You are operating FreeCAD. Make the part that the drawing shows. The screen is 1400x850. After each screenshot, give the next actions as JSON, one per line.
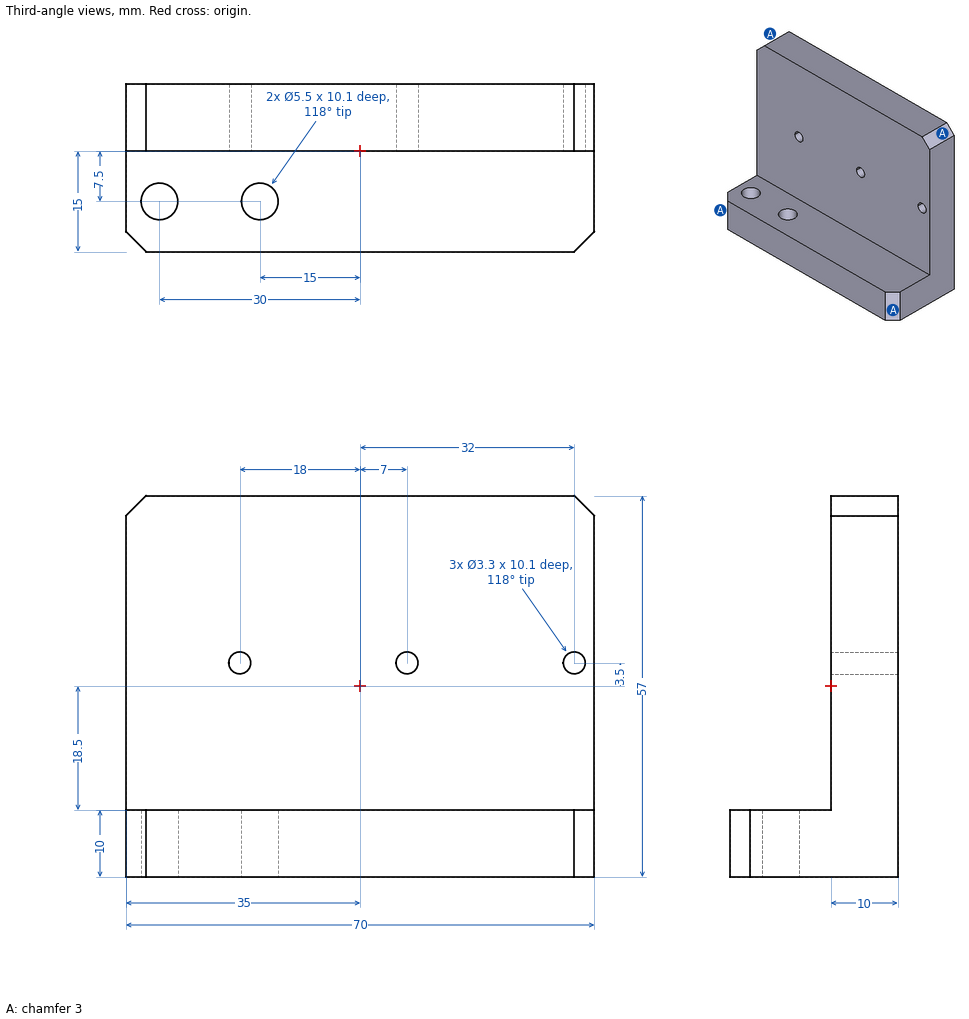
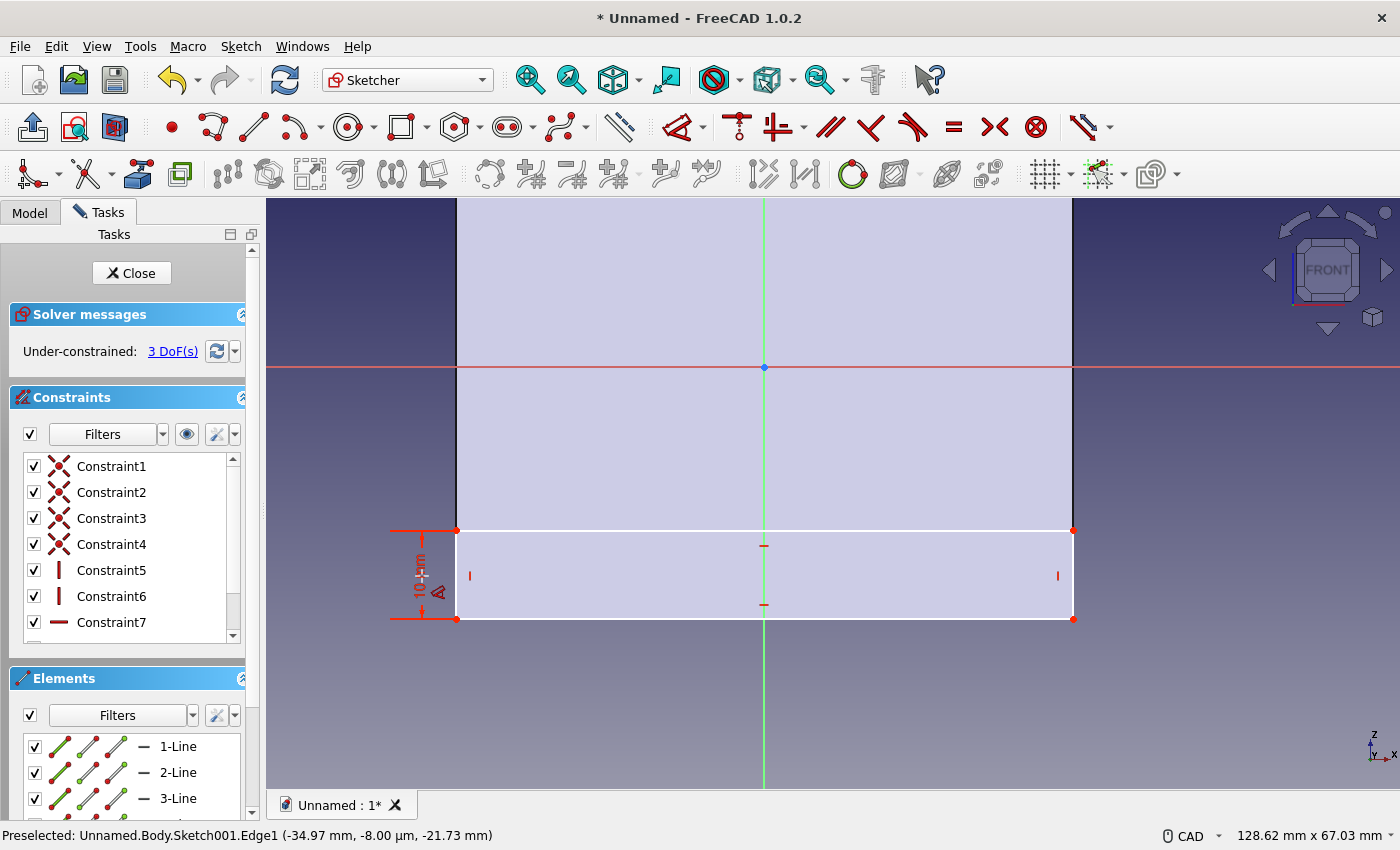
{"action": "left_click", "coordinate": [641, 619]}
{"action": "left_click", "coordinate": [623, 653]}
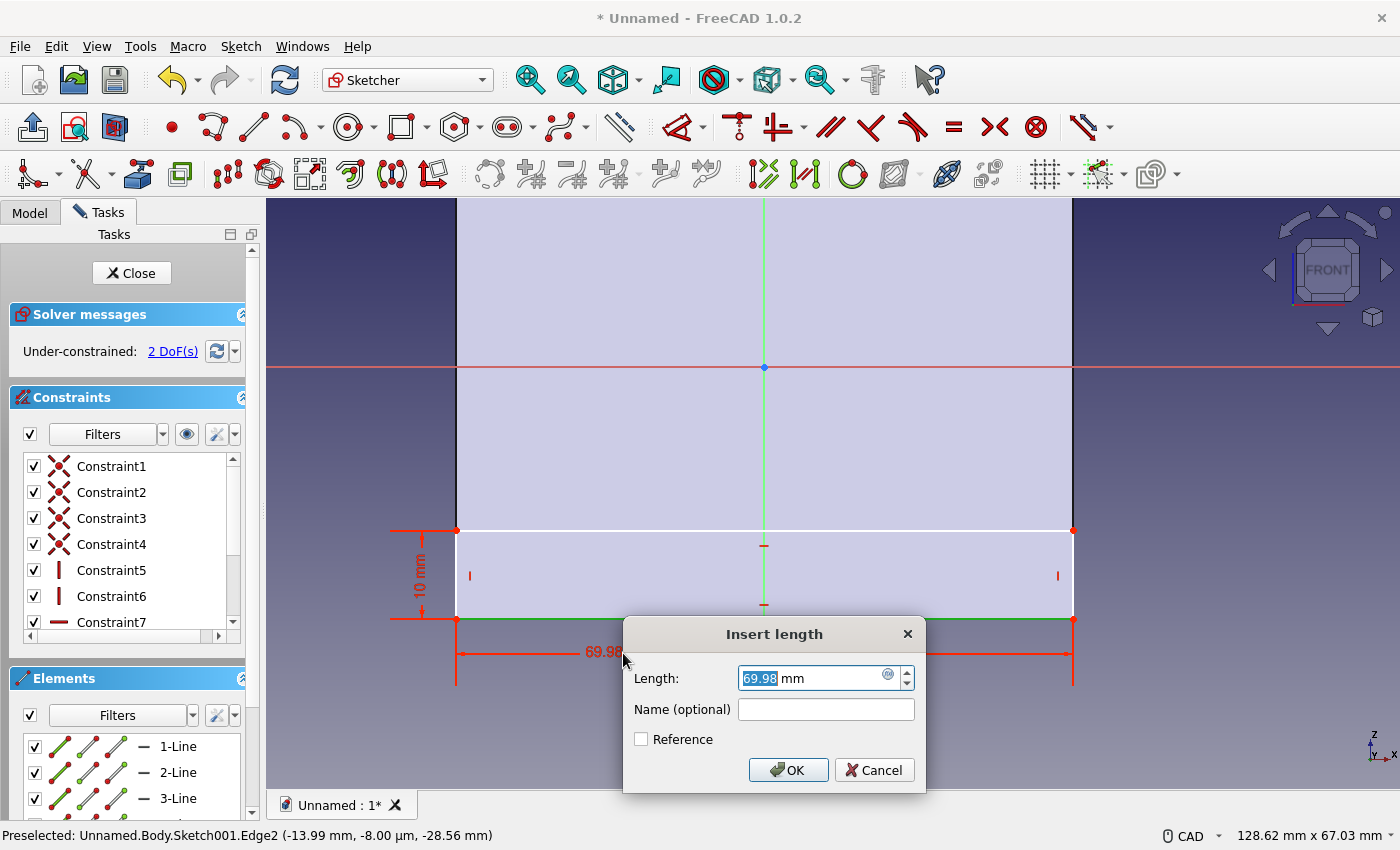
{"action": "type", "text": "70"}
{"action": "key", "text": "Return"}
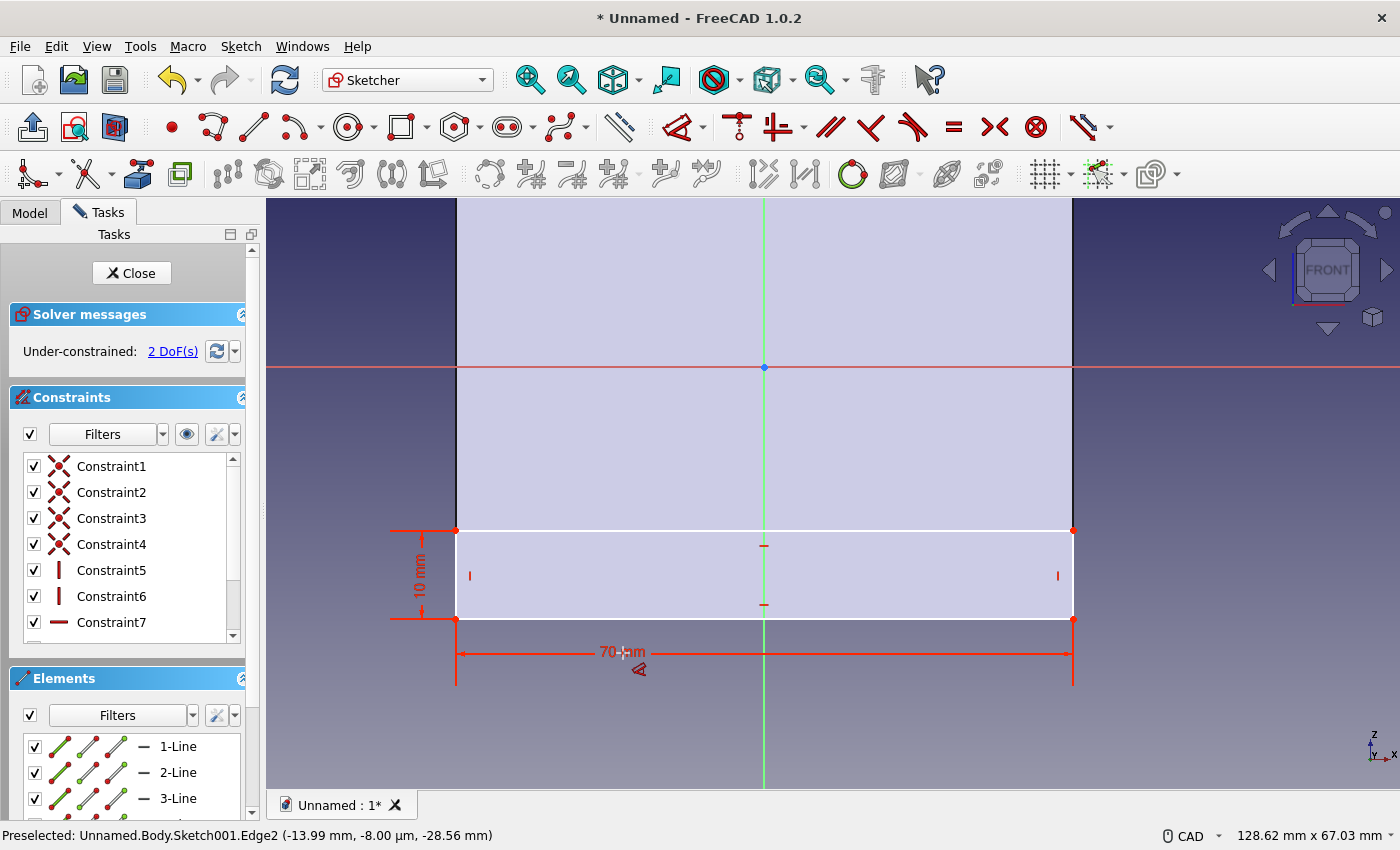
{"action": "left_click", "coordinate": [456, 531]}
{"action": "left_click", "coordinate": [610, 333]}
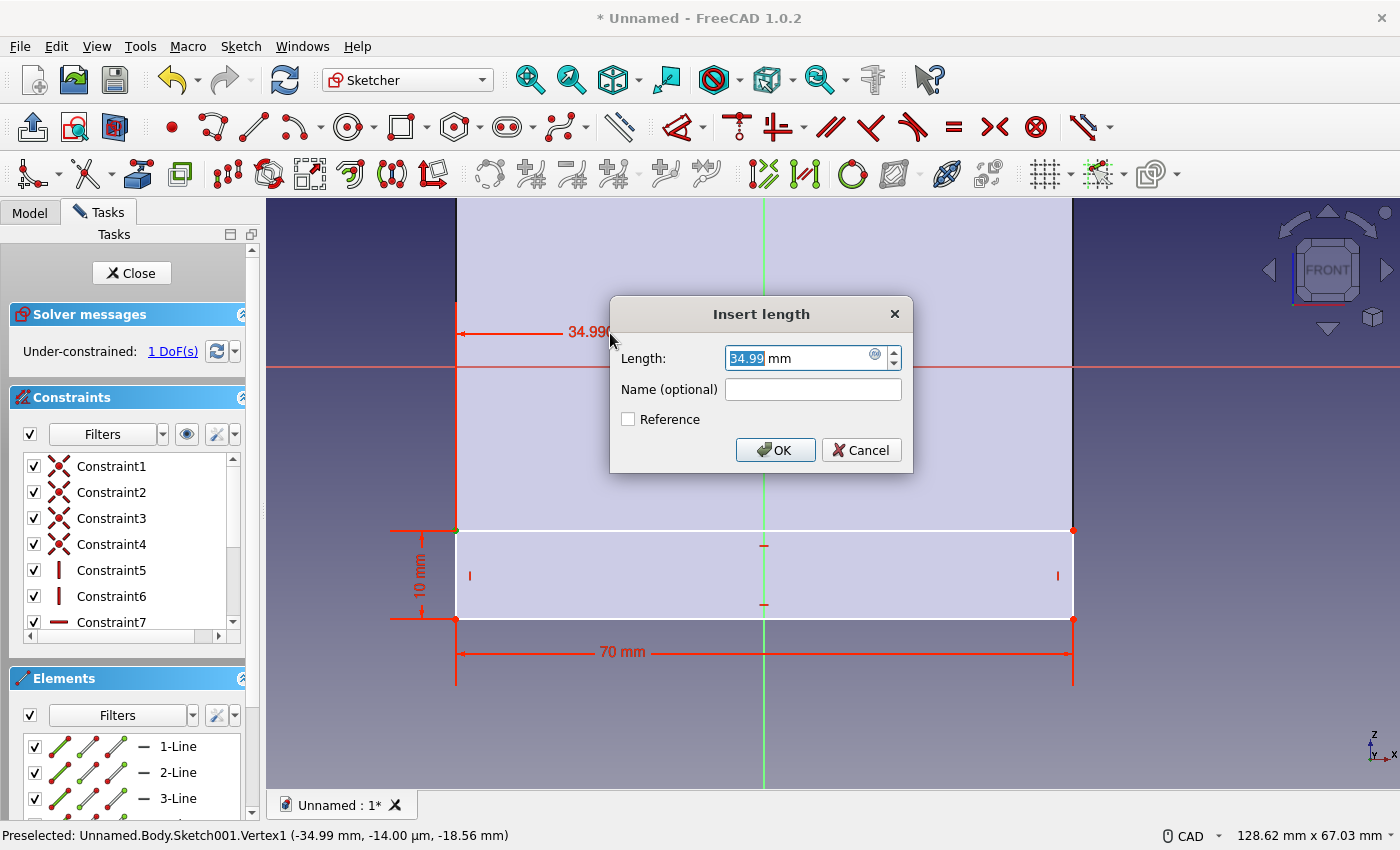
{"action": "type", "text": "35"}
{"action": "key", "text": "Return"}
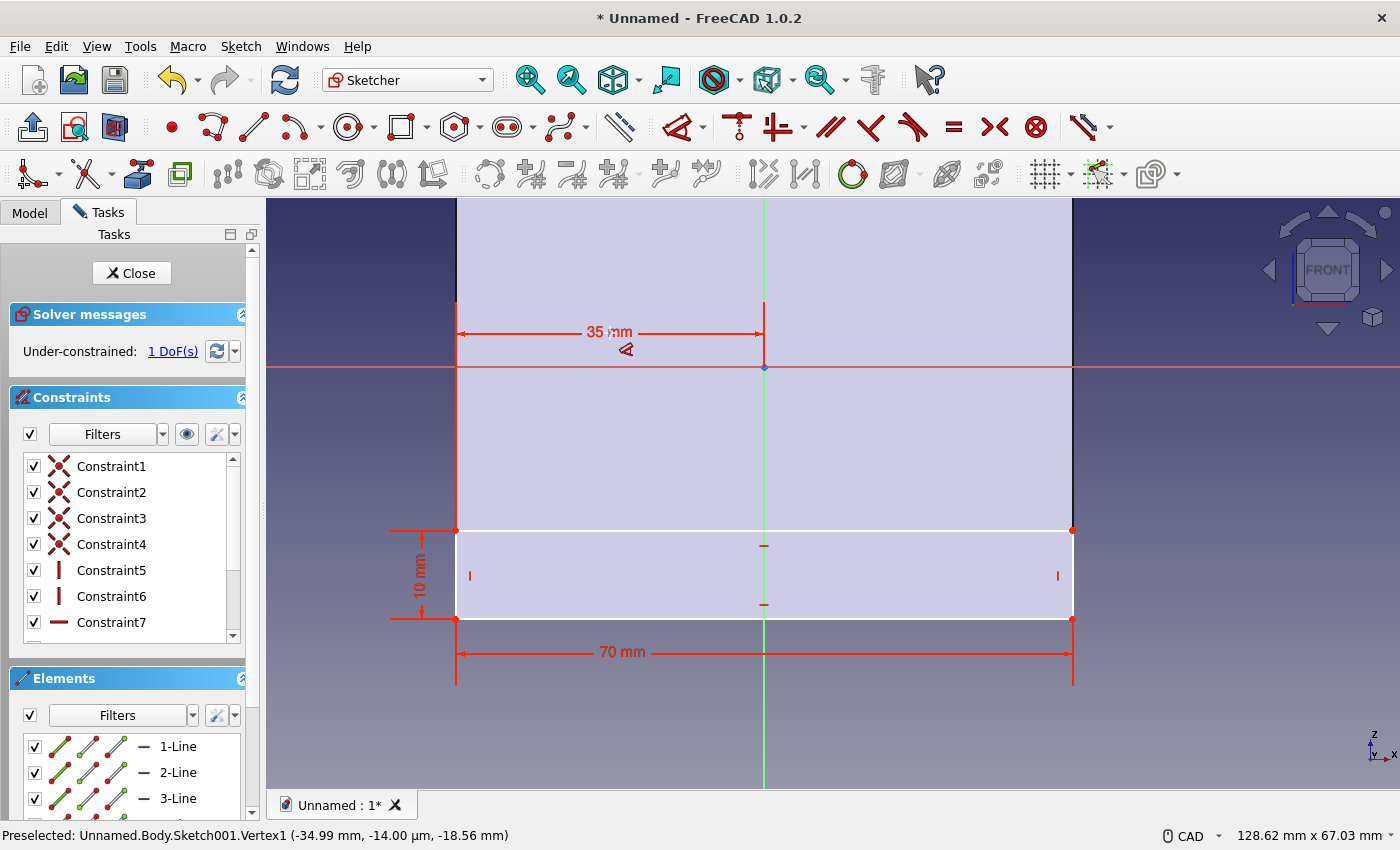
{"action": "left_click", "coordinate": [456, 531]}
{"action": "left_click", "coordinate": [422, 449]}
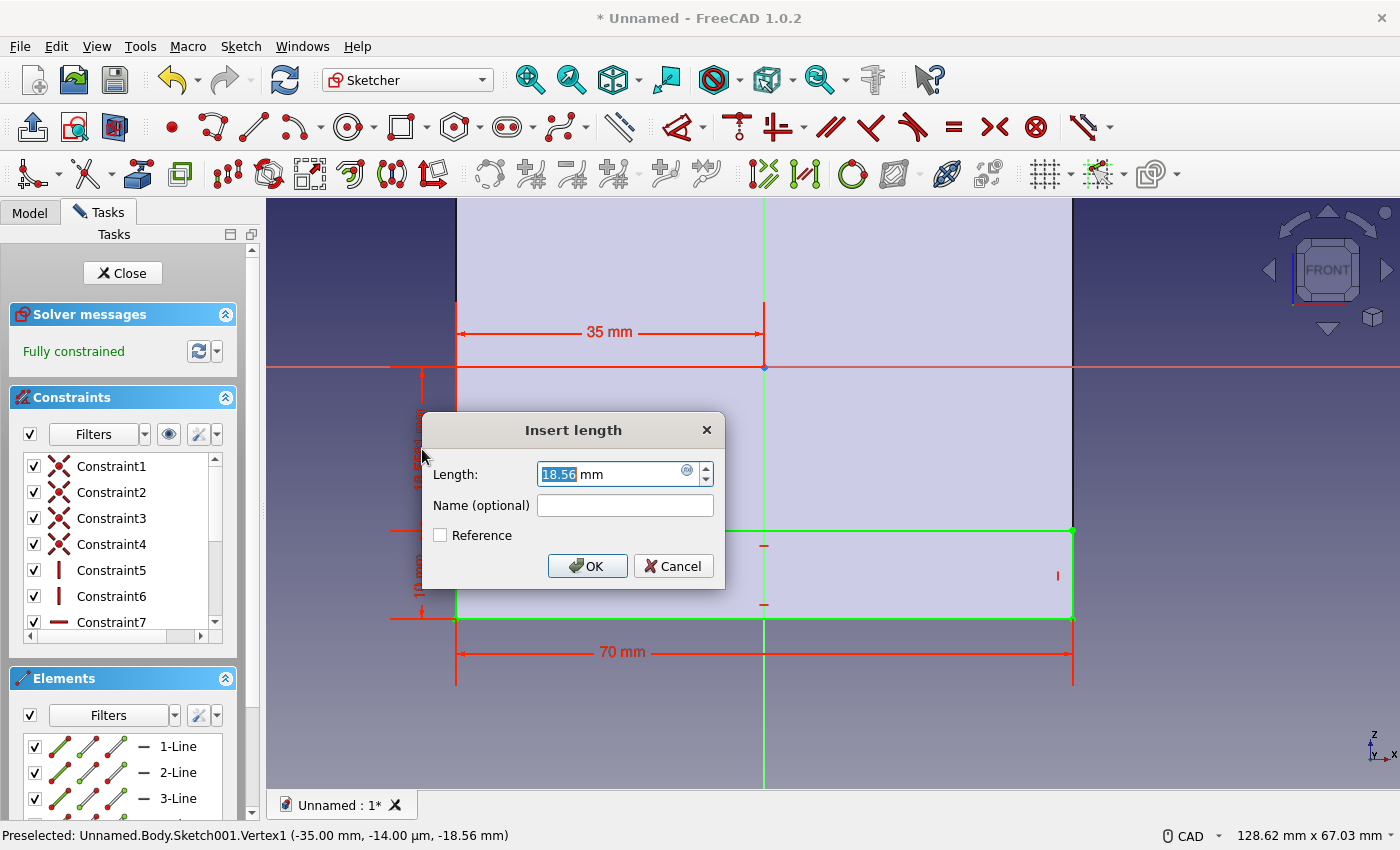
{"action": "type", "text": "18.5"}
{"action": "key", "text": "Return"}
{"action": "key", "text": "Escape"}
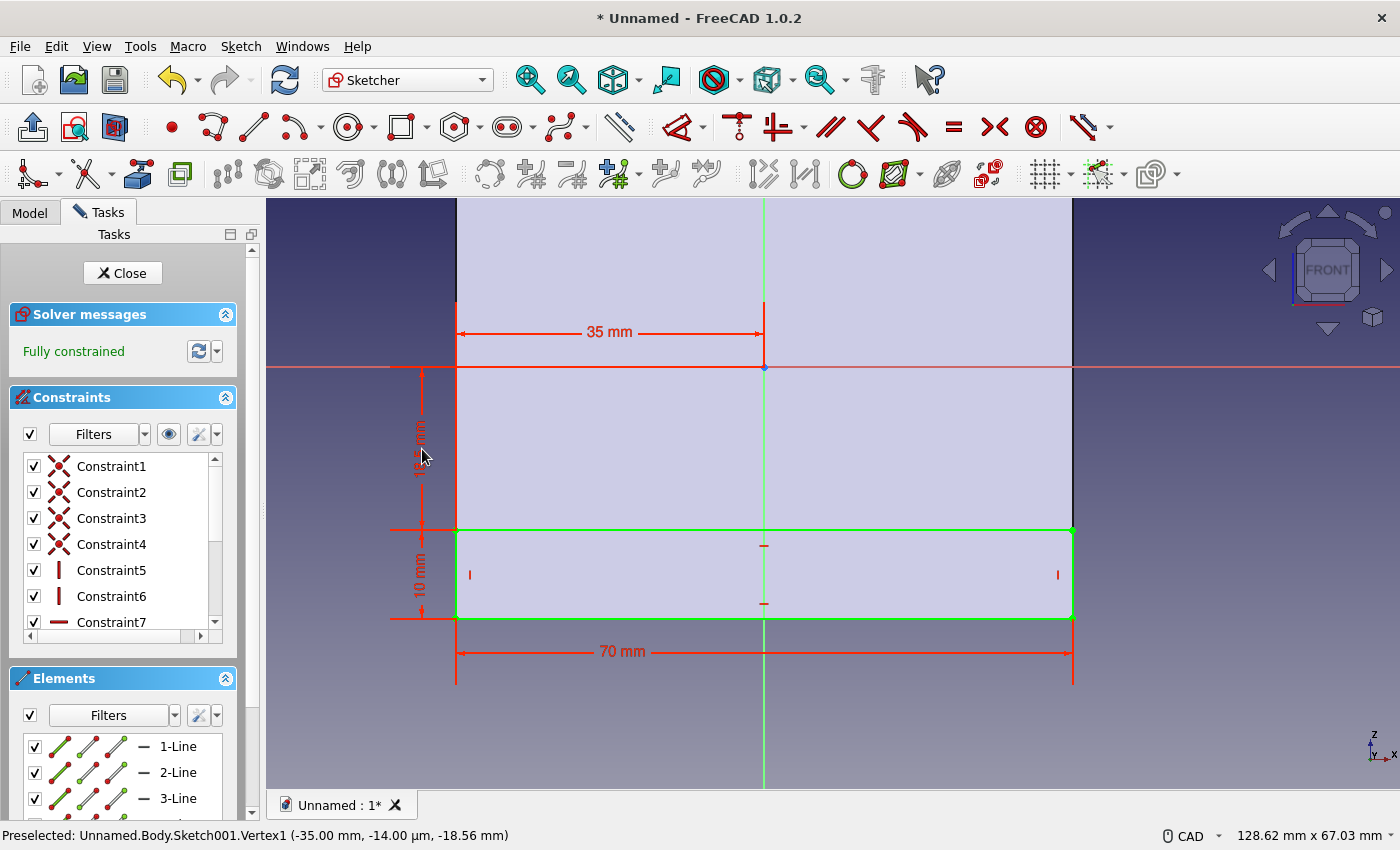
{"action": "left_click", "coordinate": [123, 273]}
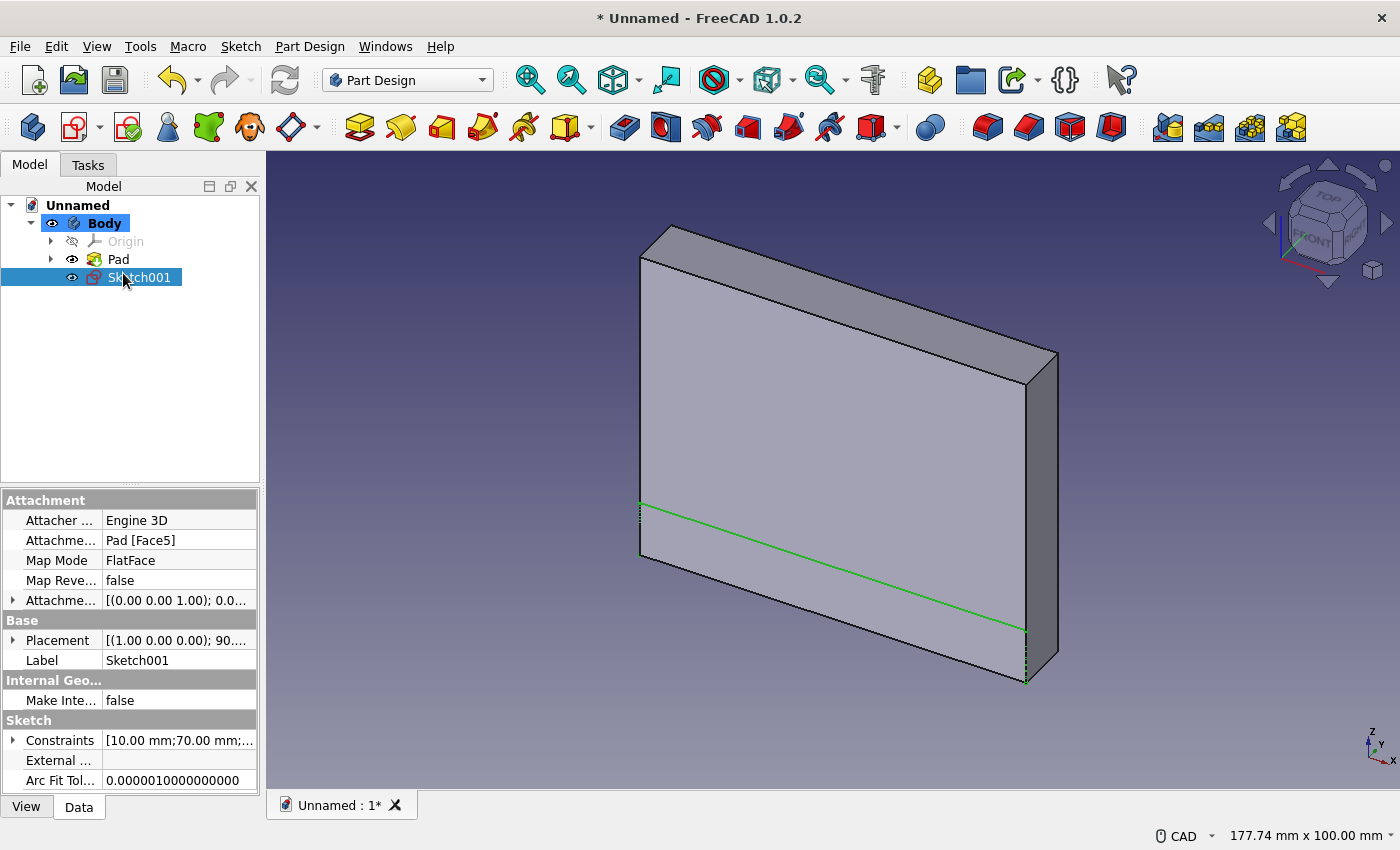
{"action": "left_click", "coordinate": [360, 128]}